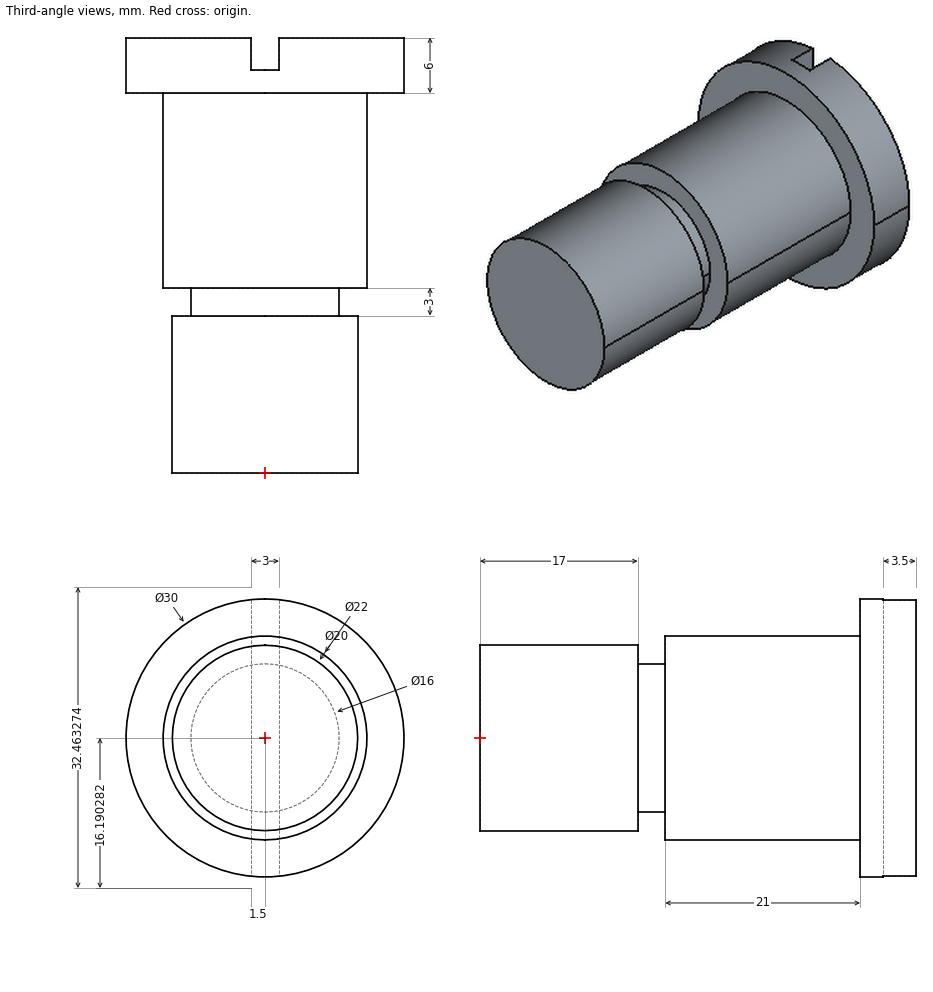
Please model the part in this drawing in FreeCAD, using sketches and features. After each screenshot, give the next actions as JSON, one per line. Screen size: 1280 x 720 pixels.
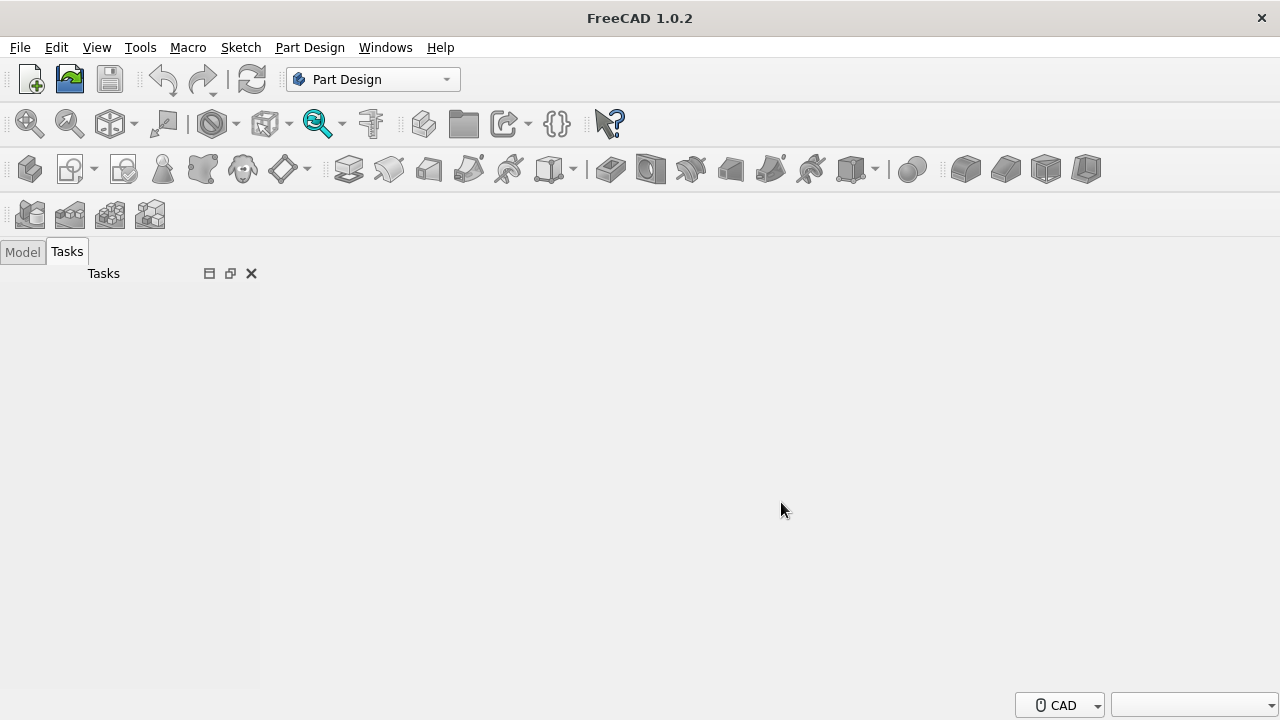
{"action": "left_click", "coordinate": [30, 80]}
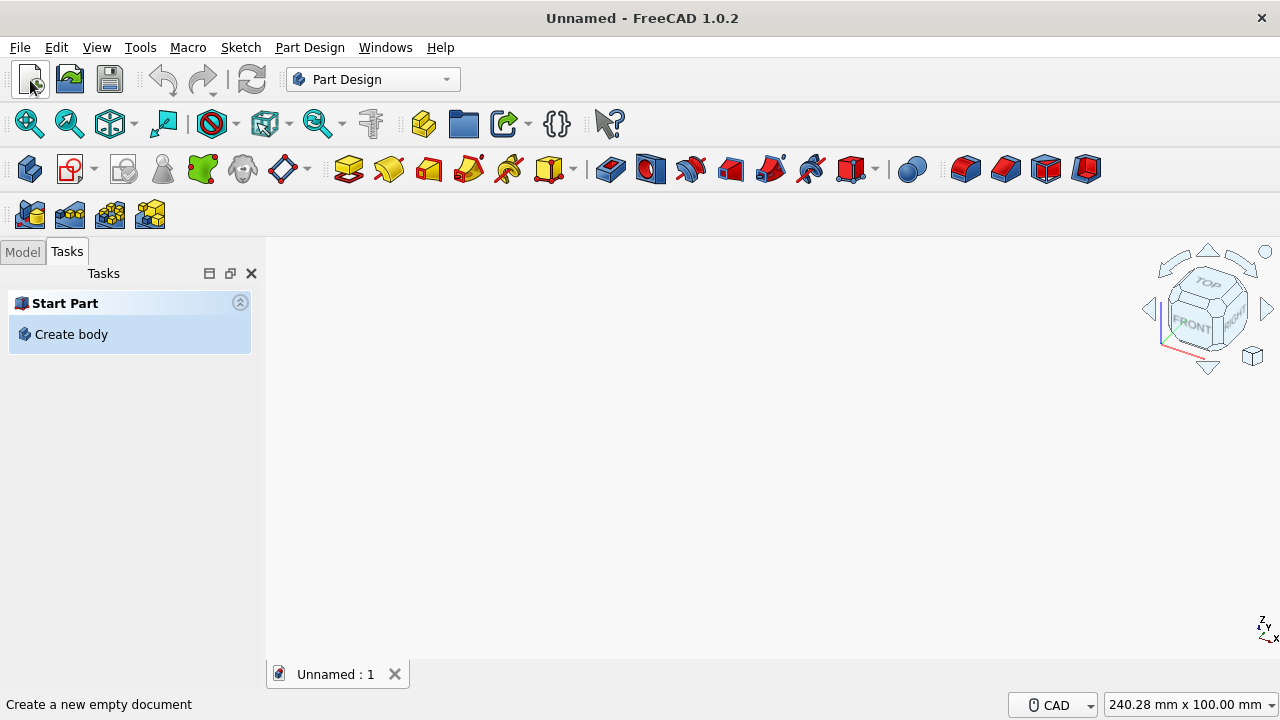
{"action": "left_click", "coordinate": [70, 170]}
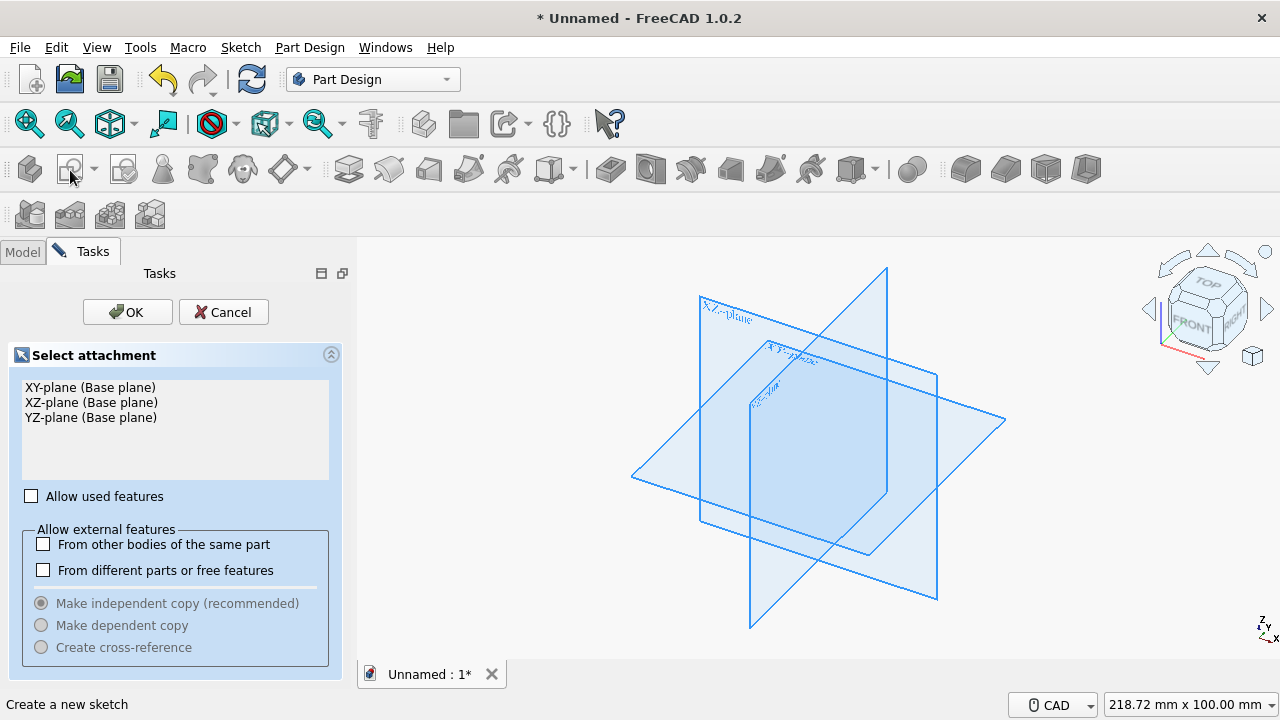
{"action": "left_click", "coordinate": [82, 402]}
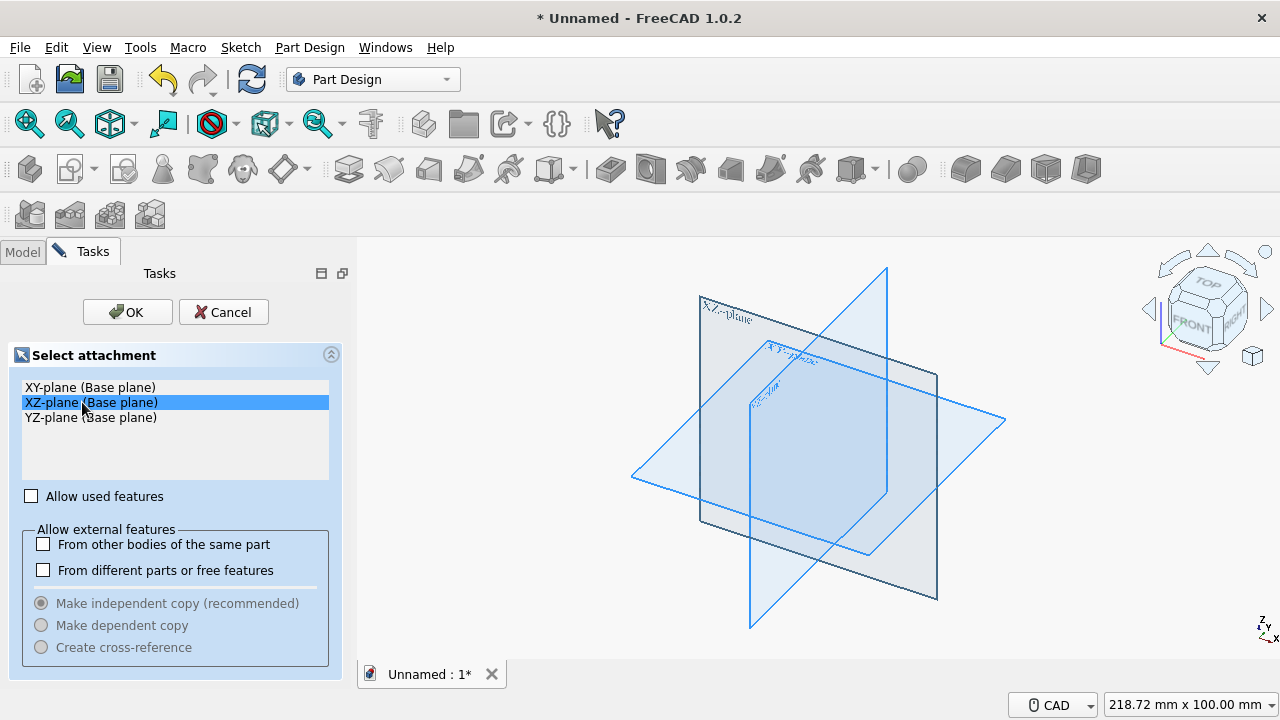
{"action": "left_click", "coordinate": [128, 312]}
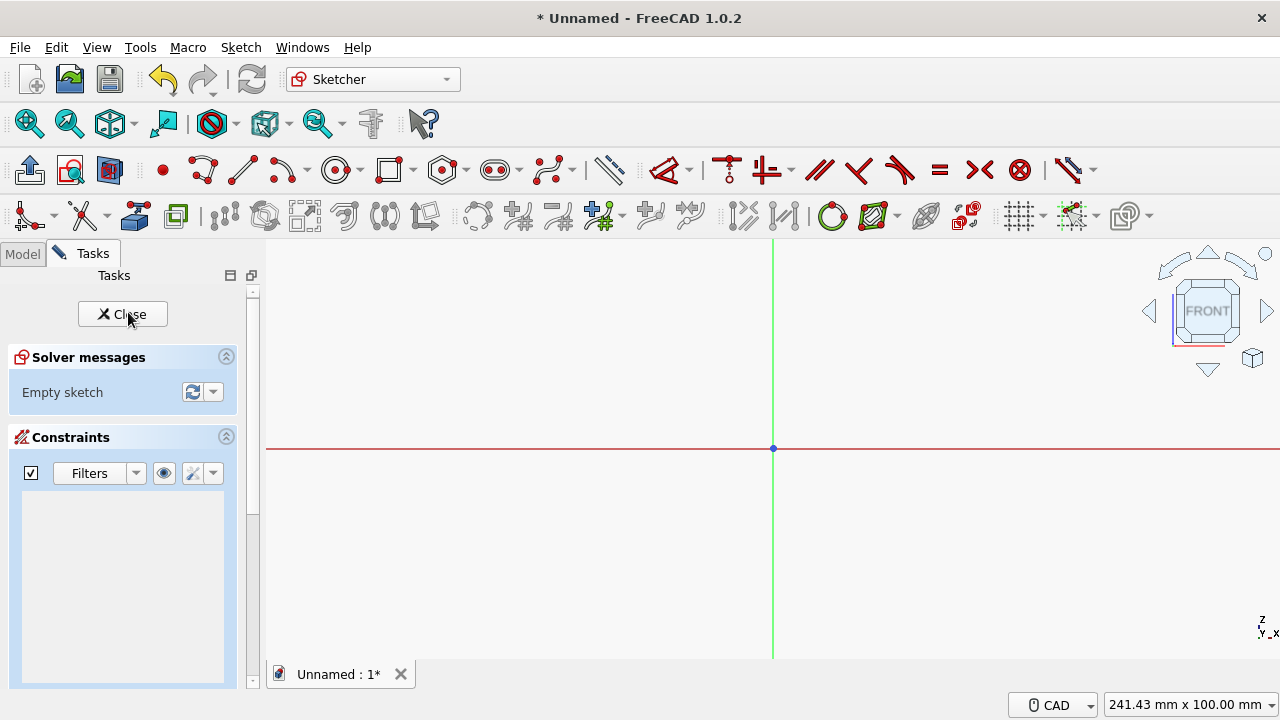
{"action": "scroll", "coordinate": [803, 449], "scroll_direction": "up", "scroll_amount": 6}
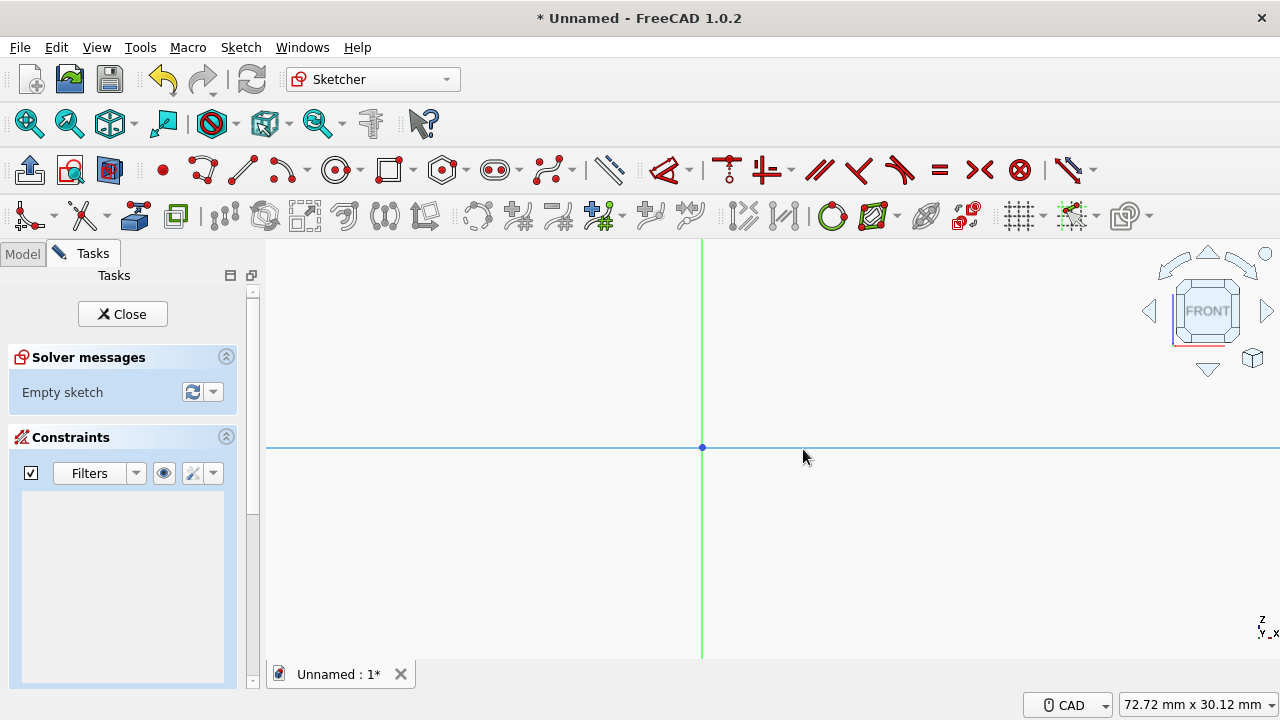
{"action": "left_click", "coordinate": [336, 170]}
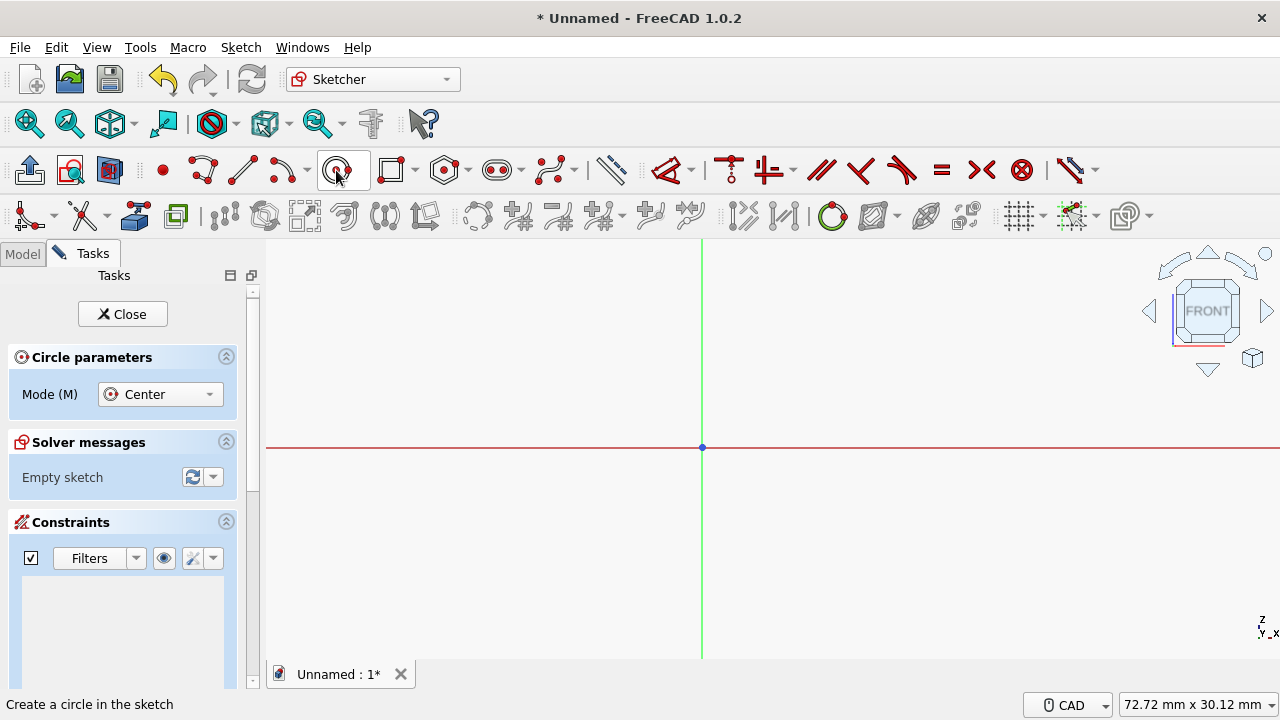
{"action": "left_click", "coordinate": [702, 448]}
{"action": "mouse_move", "coordinate": [801, 349]}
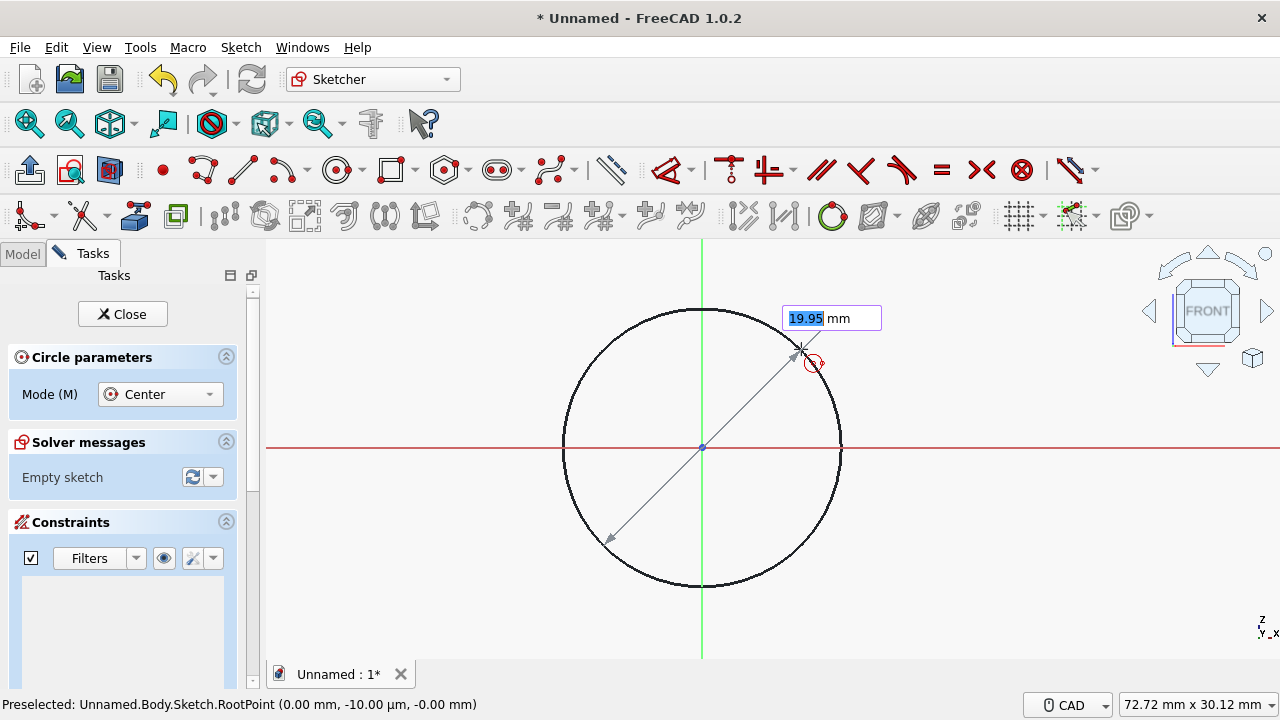
{"action": "type", "text": "20"}
{"action": "key", "text": "Return"}
{"action": "key", "text": "Escape"}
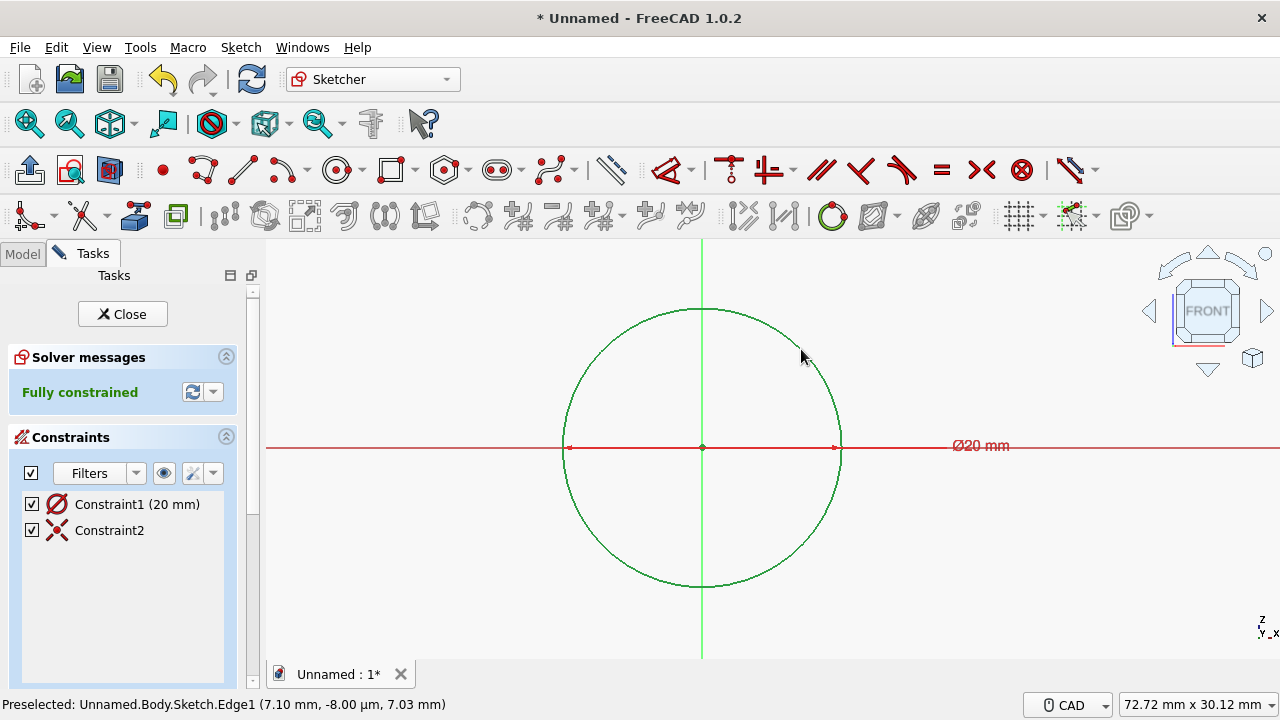
{"action": "left_click", "coordinate": [123, 314]}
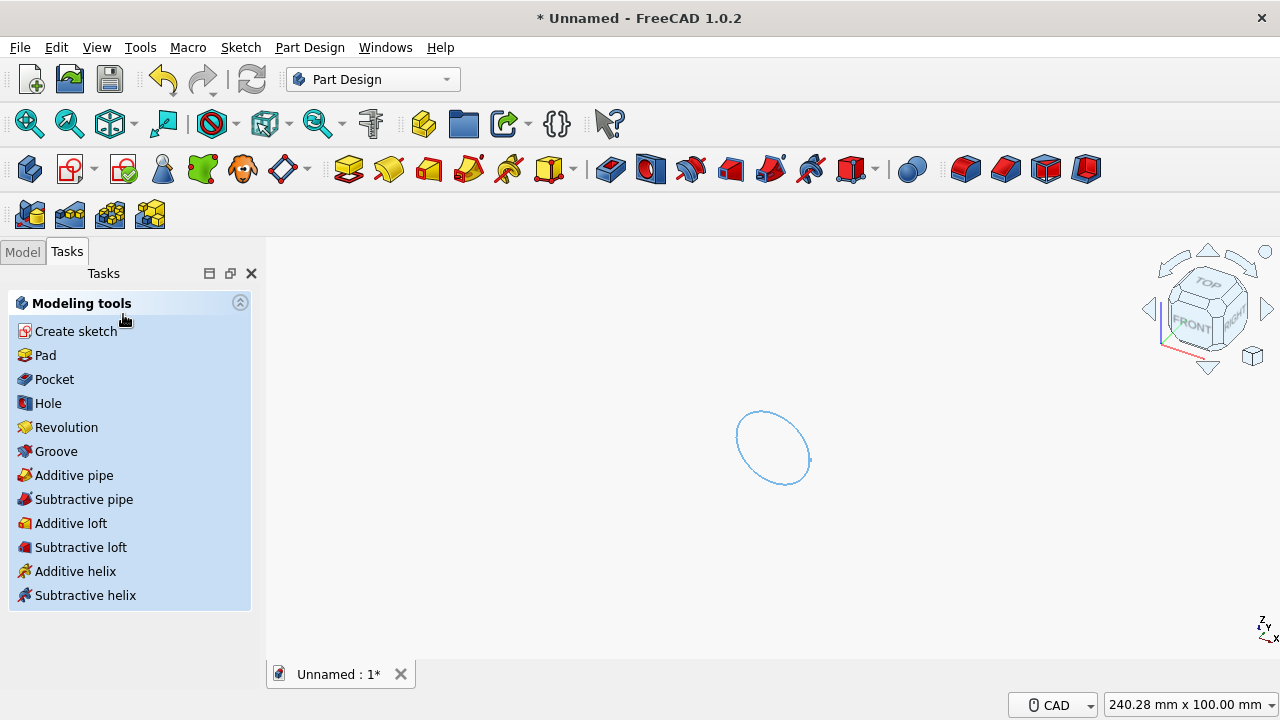
{"action": "left_click", "coordinate": [350, 170]}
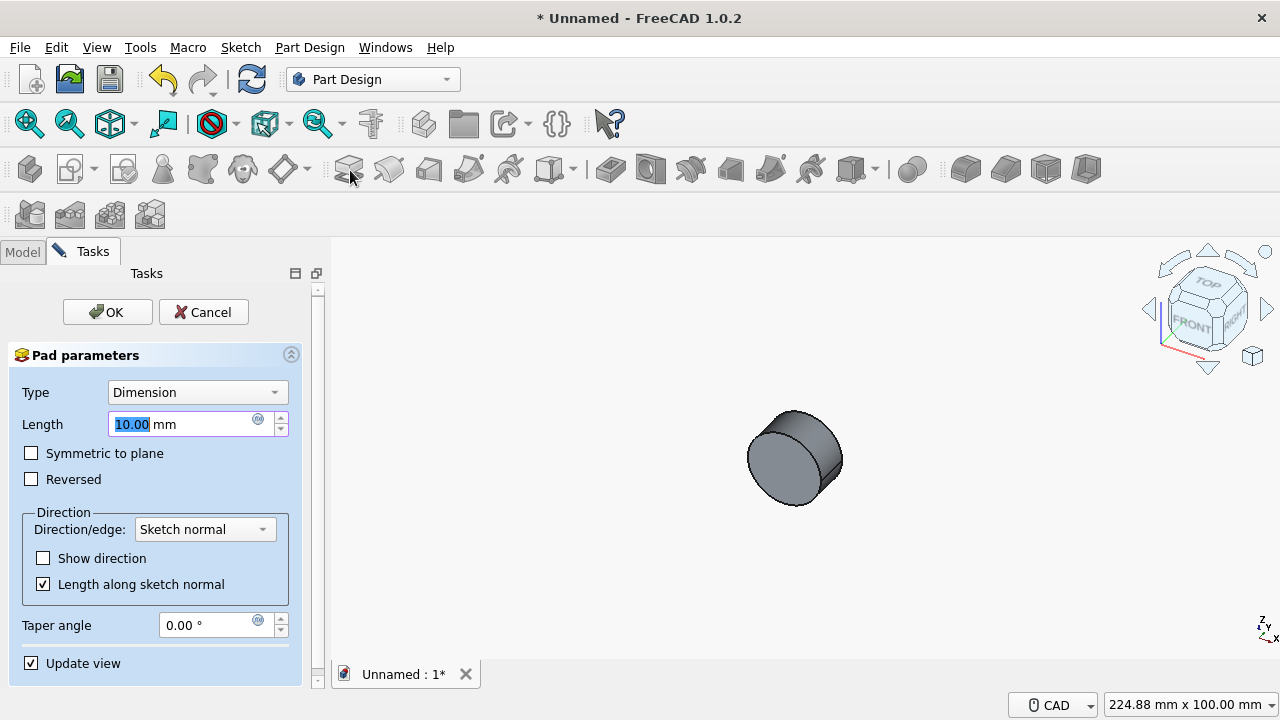
{"action": "type", "text": "17"}
{"action": "key", "text": "Tab"}